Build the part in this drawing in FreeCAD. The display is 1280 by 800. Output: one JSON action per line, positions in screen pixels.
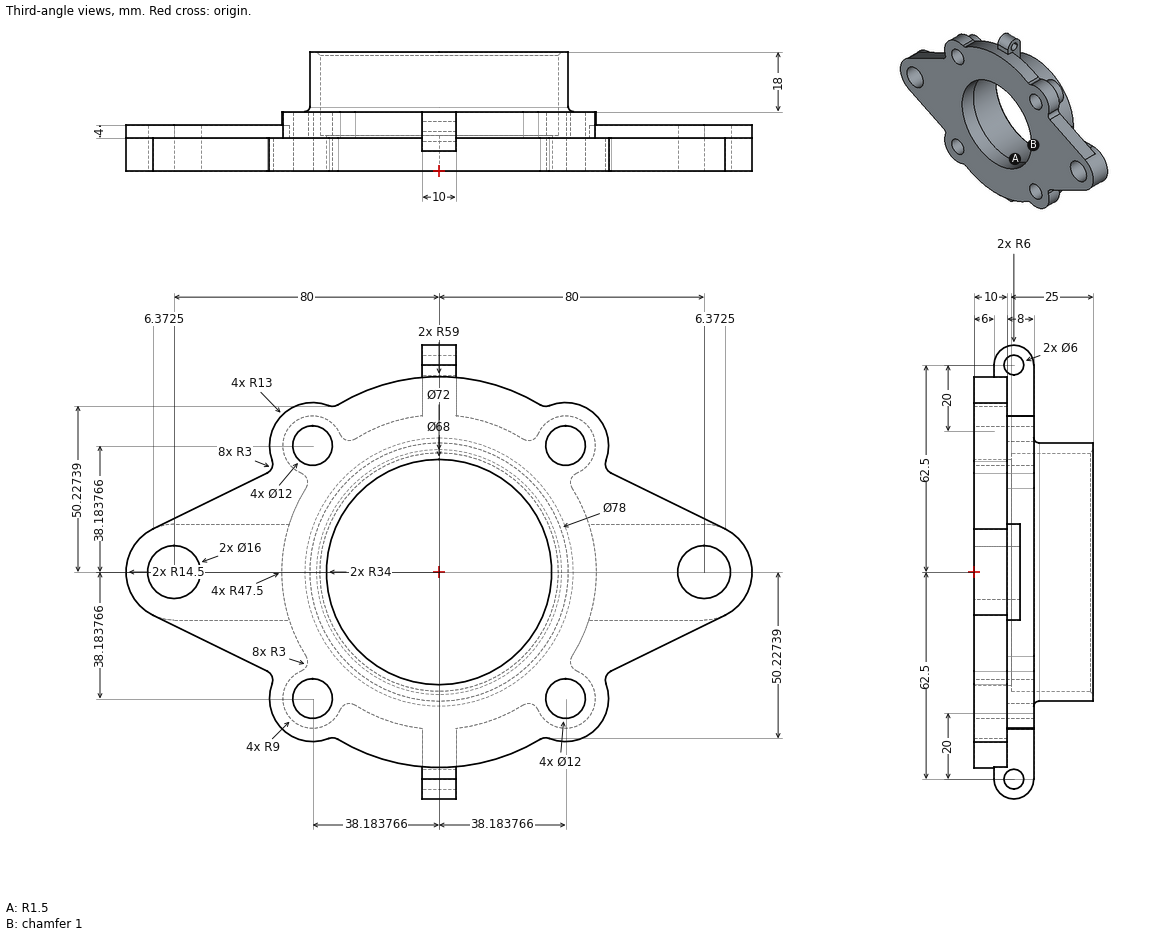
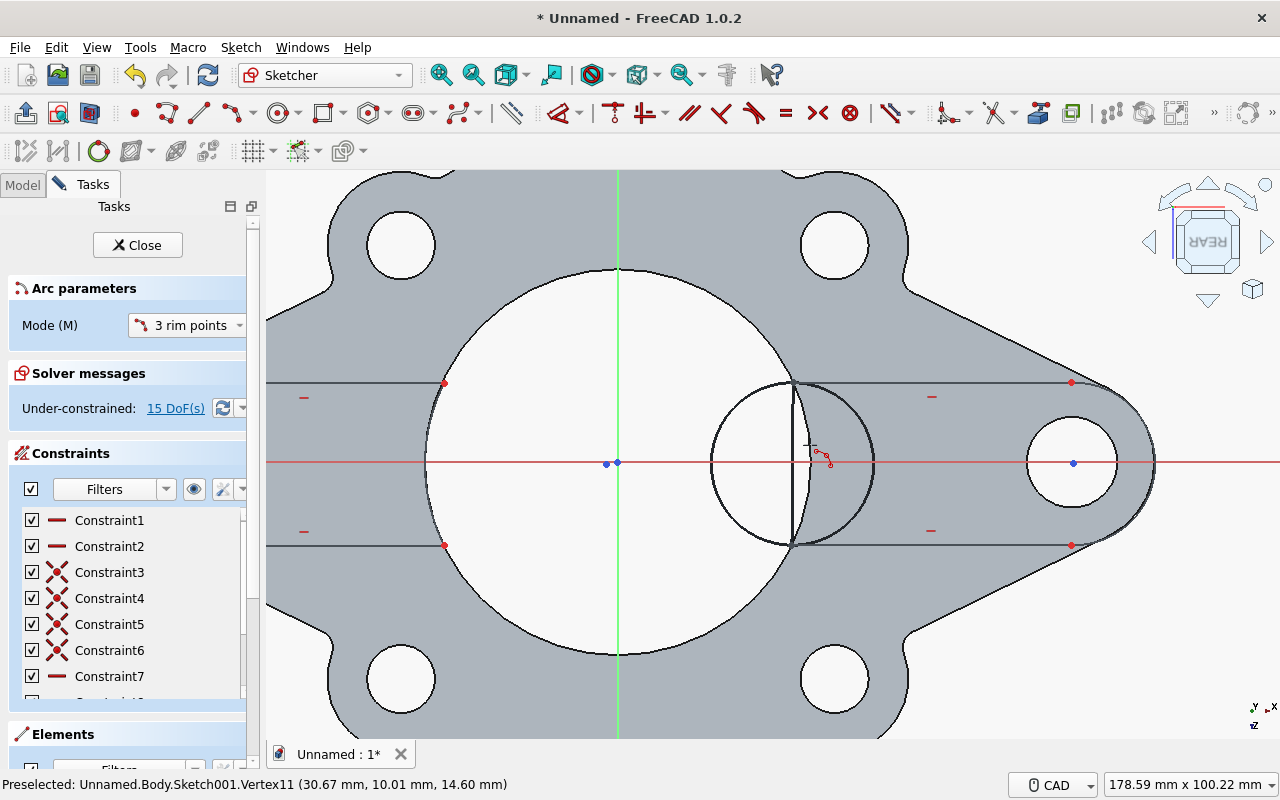
{"action": "left_click", "coordinate": [810, 445]}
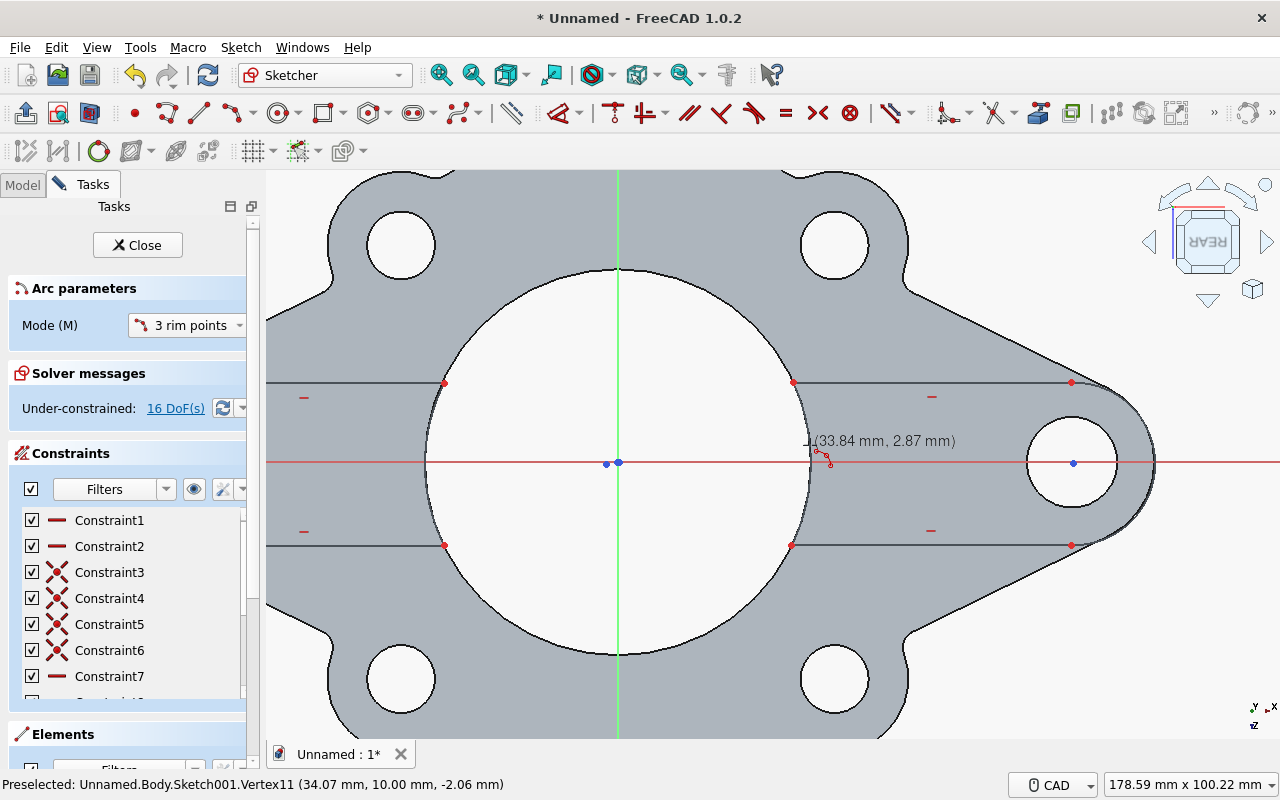
{"action": "left_click", "coordinate": [278, 114]}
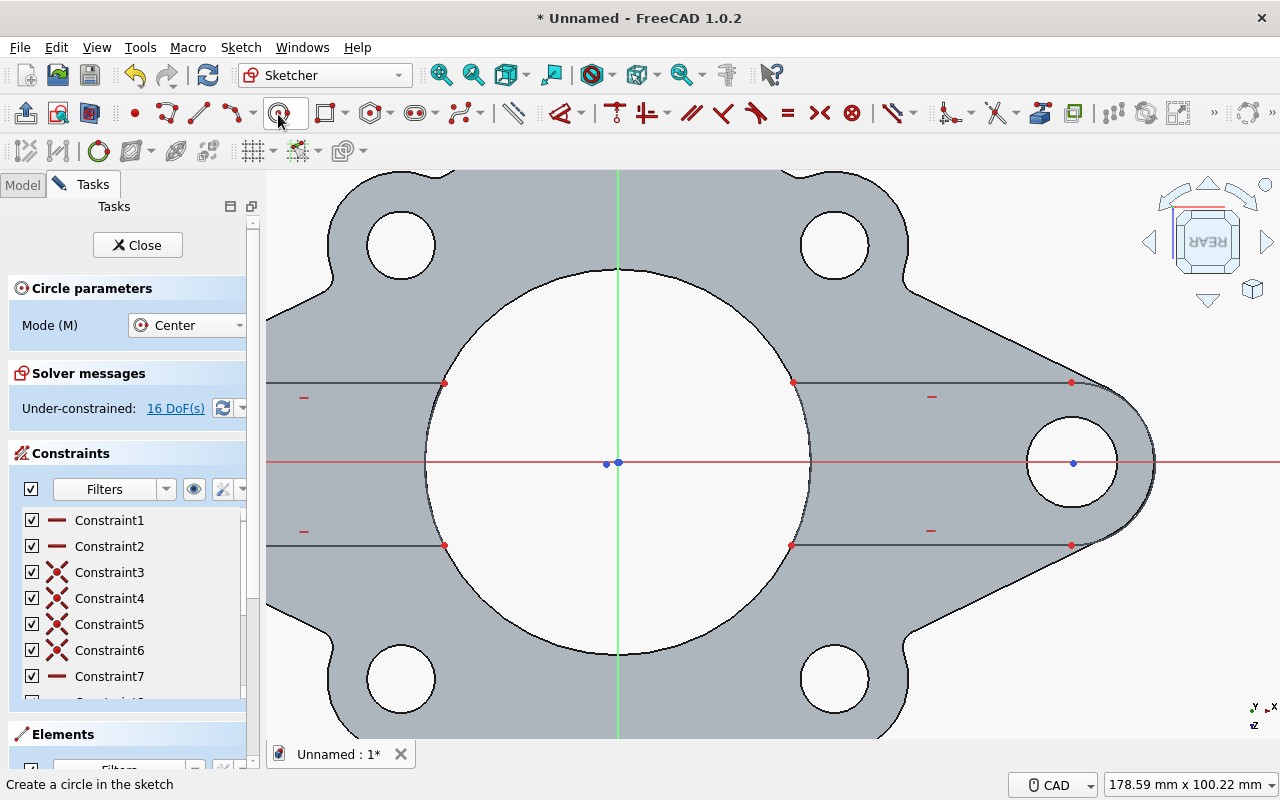
{"action": "scroll", "coordinate": [810, 445], "scroll_direction": "down", "scroll_amount": 3}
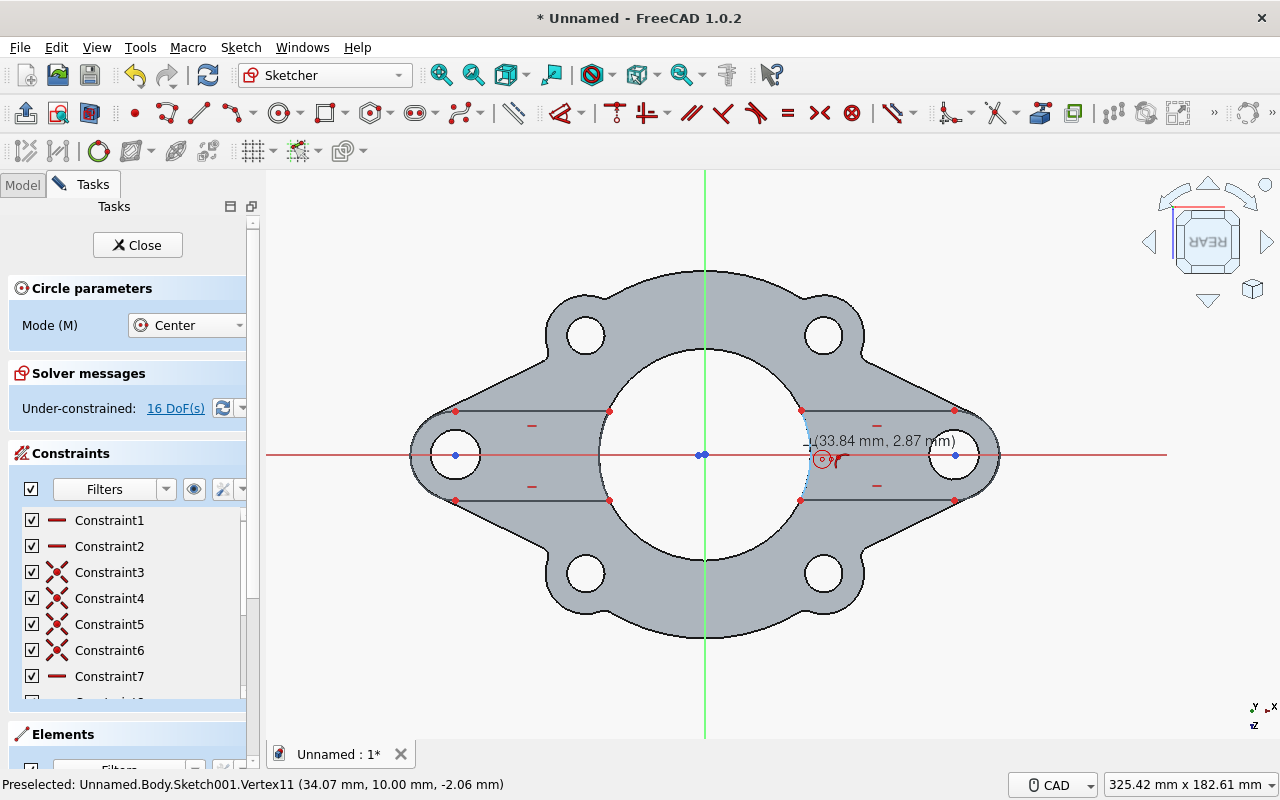
{"action": "left_click", "coordinate": [456, 455]}
{"action": "mouse_move", "coordinate": [473, 437]}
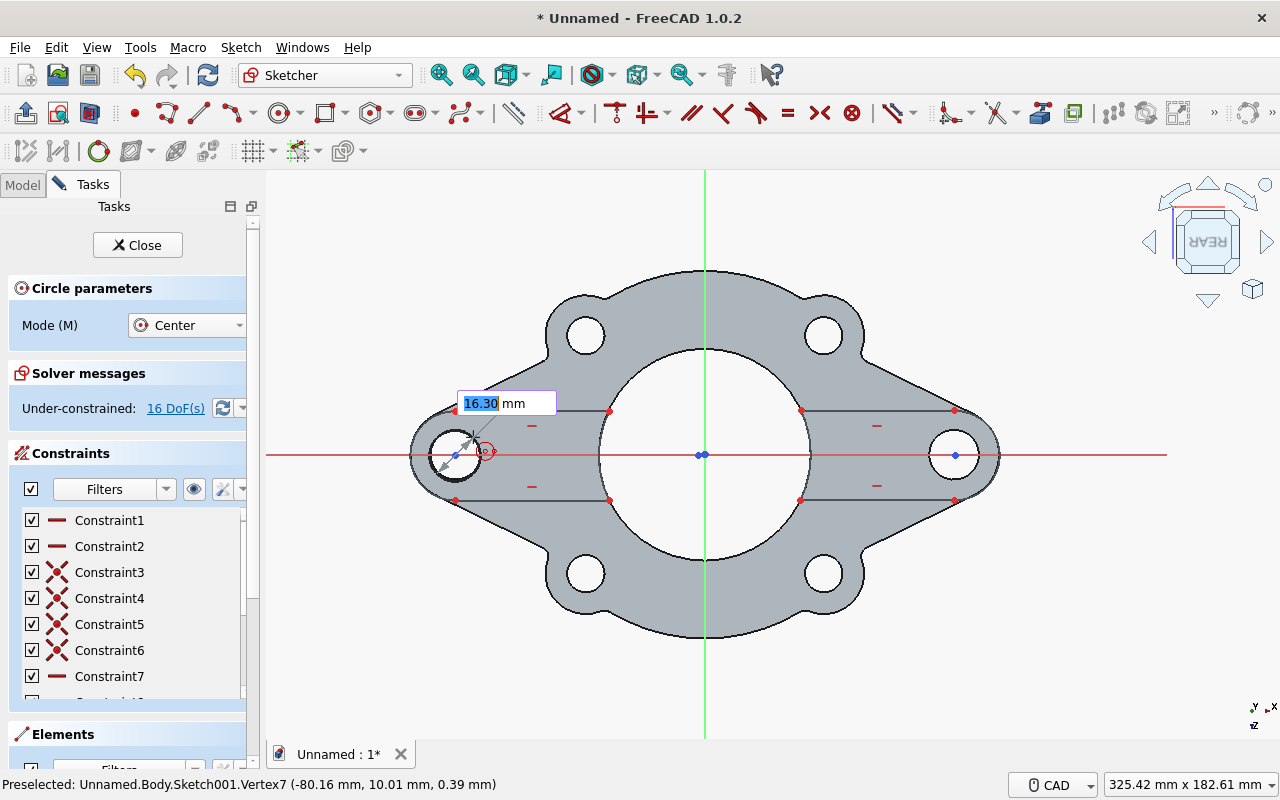
{"action": "type", "text": "16"}
{"action": "key", "text": "Return"}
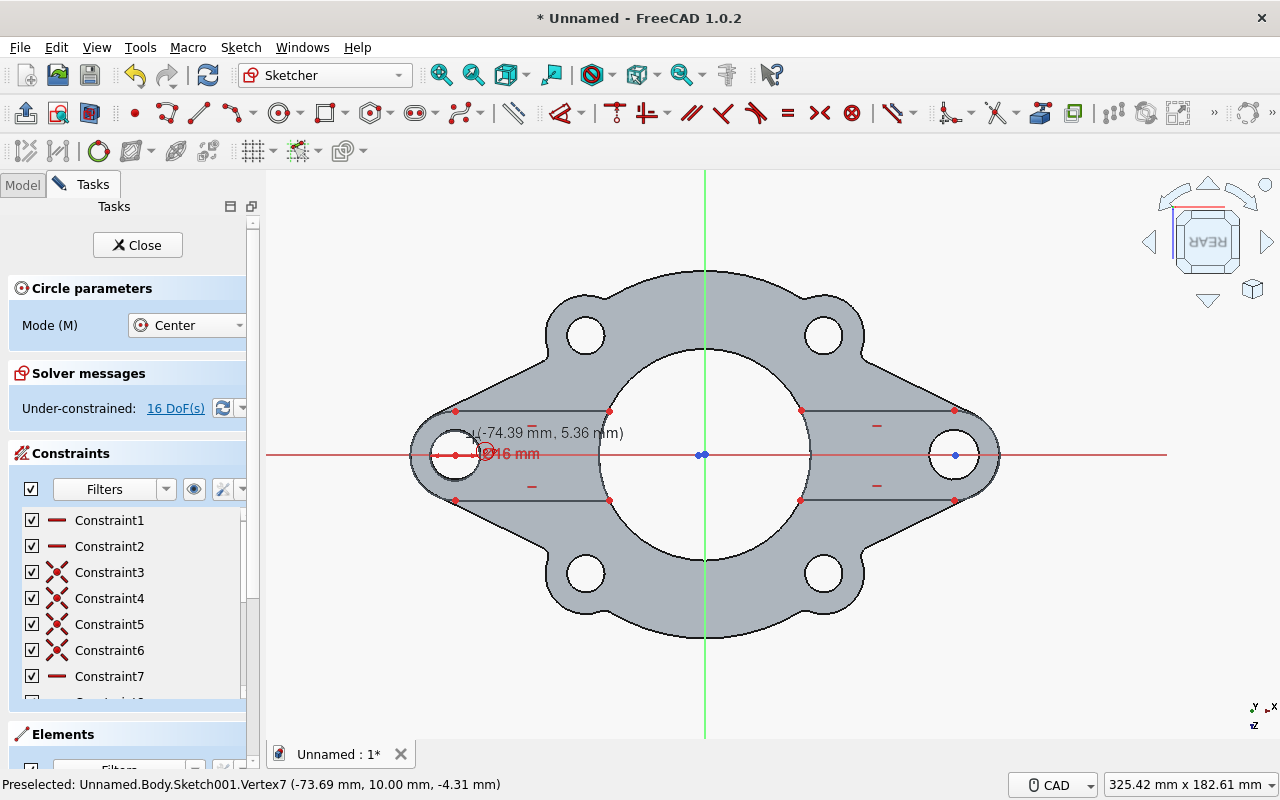
{"action": "left_click", "coordinate": [954, 455]}
{"action": "mouse_move", "coordinate": [972, 437]}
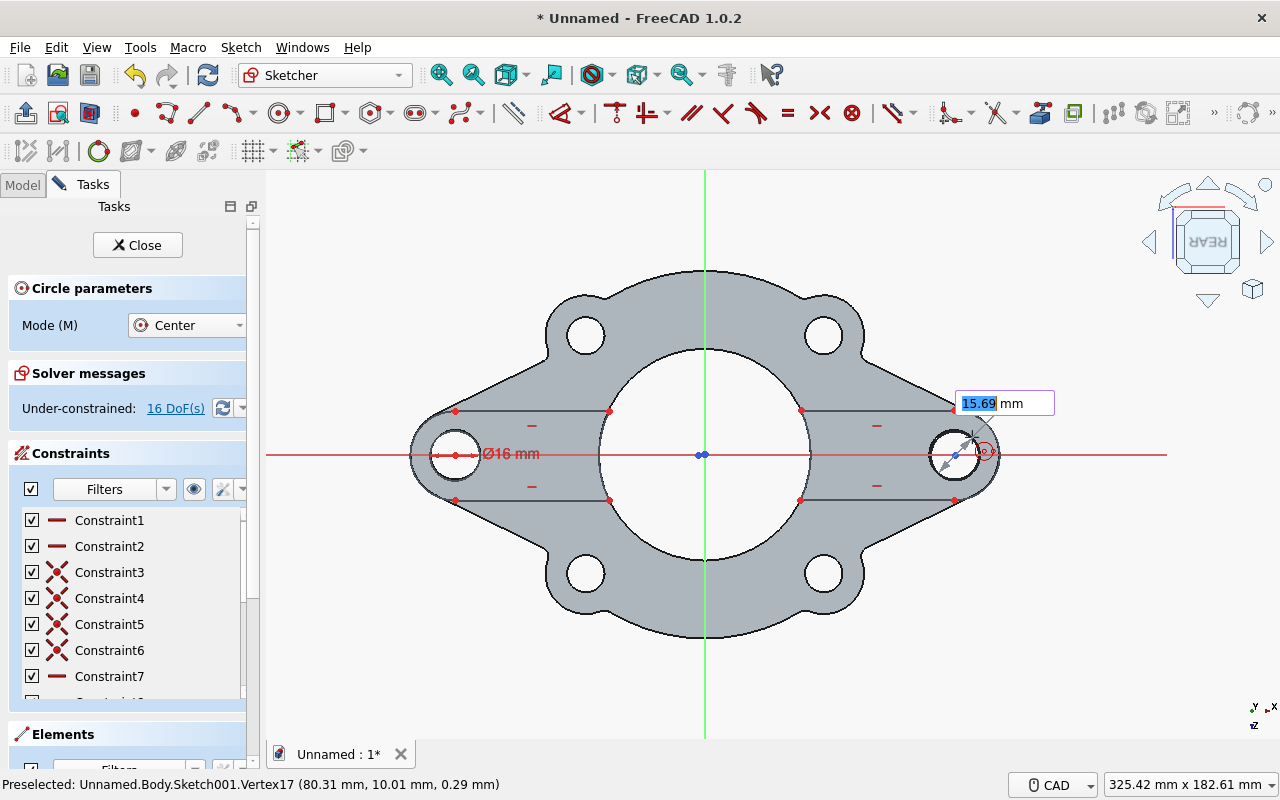
{"action": "type", "text": "16"}
{"action": "key", "text": "Return"}
{"action": "key", "text": "Escape"}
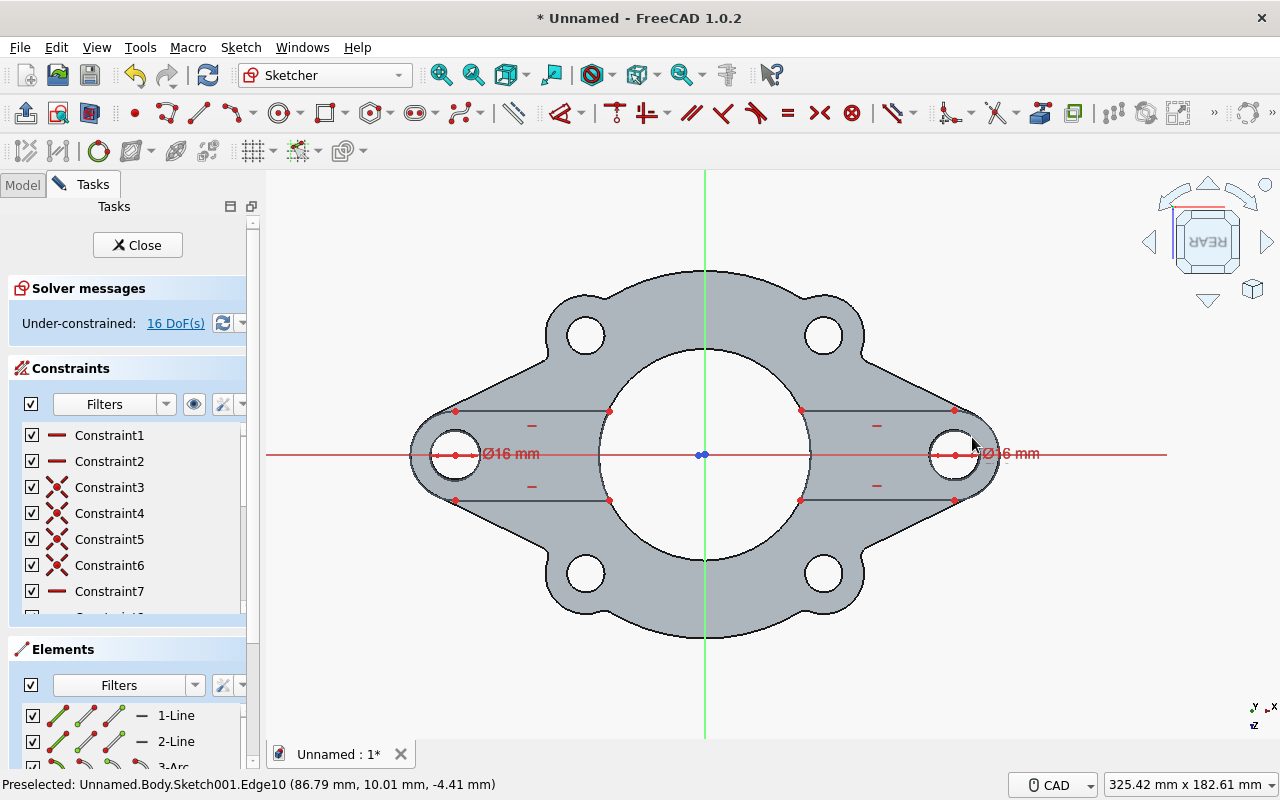
{"action": "left_click", "coordinate": [563, 411]}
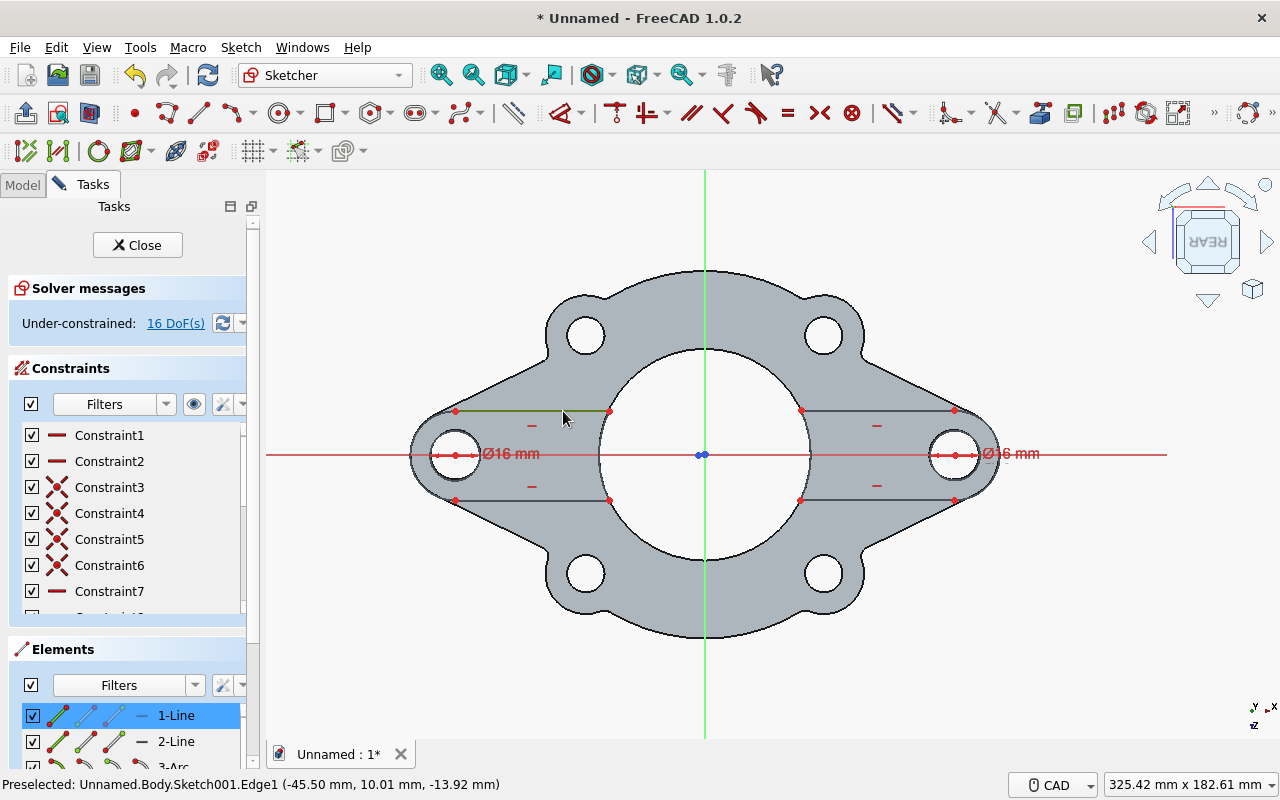
{"action": "left_click", "coordinate": [419, 430]}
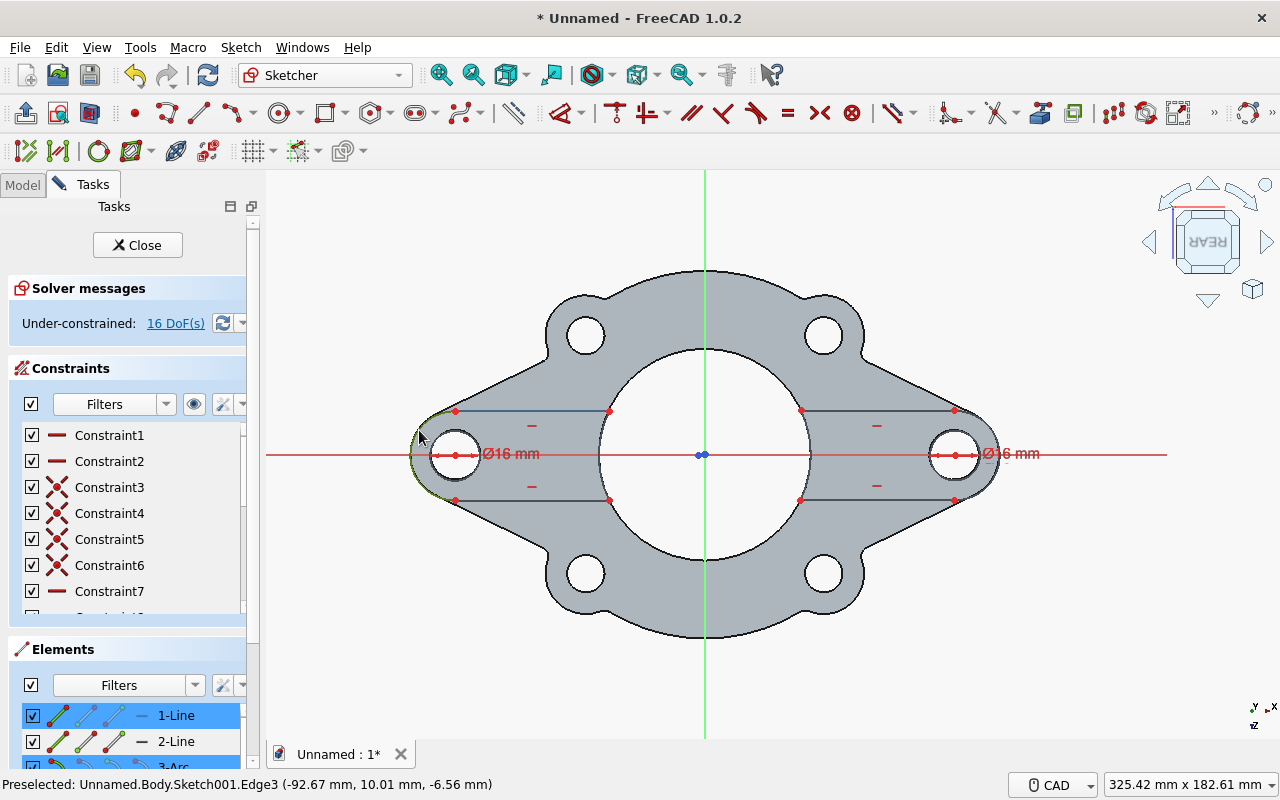
{"action": "left_click", "coordinate": [756, 114]}